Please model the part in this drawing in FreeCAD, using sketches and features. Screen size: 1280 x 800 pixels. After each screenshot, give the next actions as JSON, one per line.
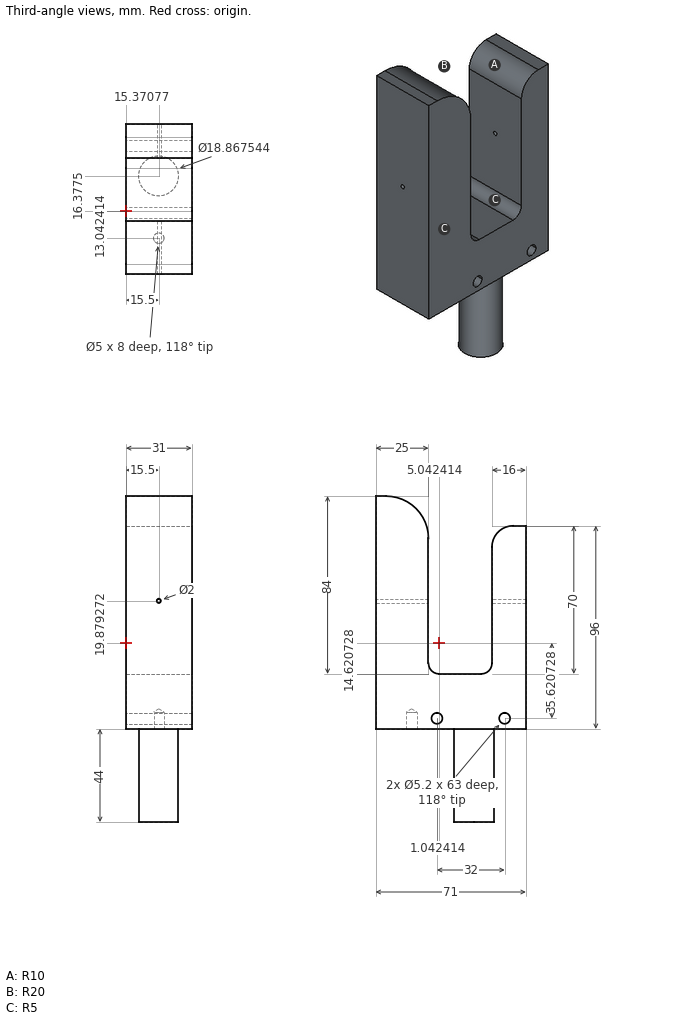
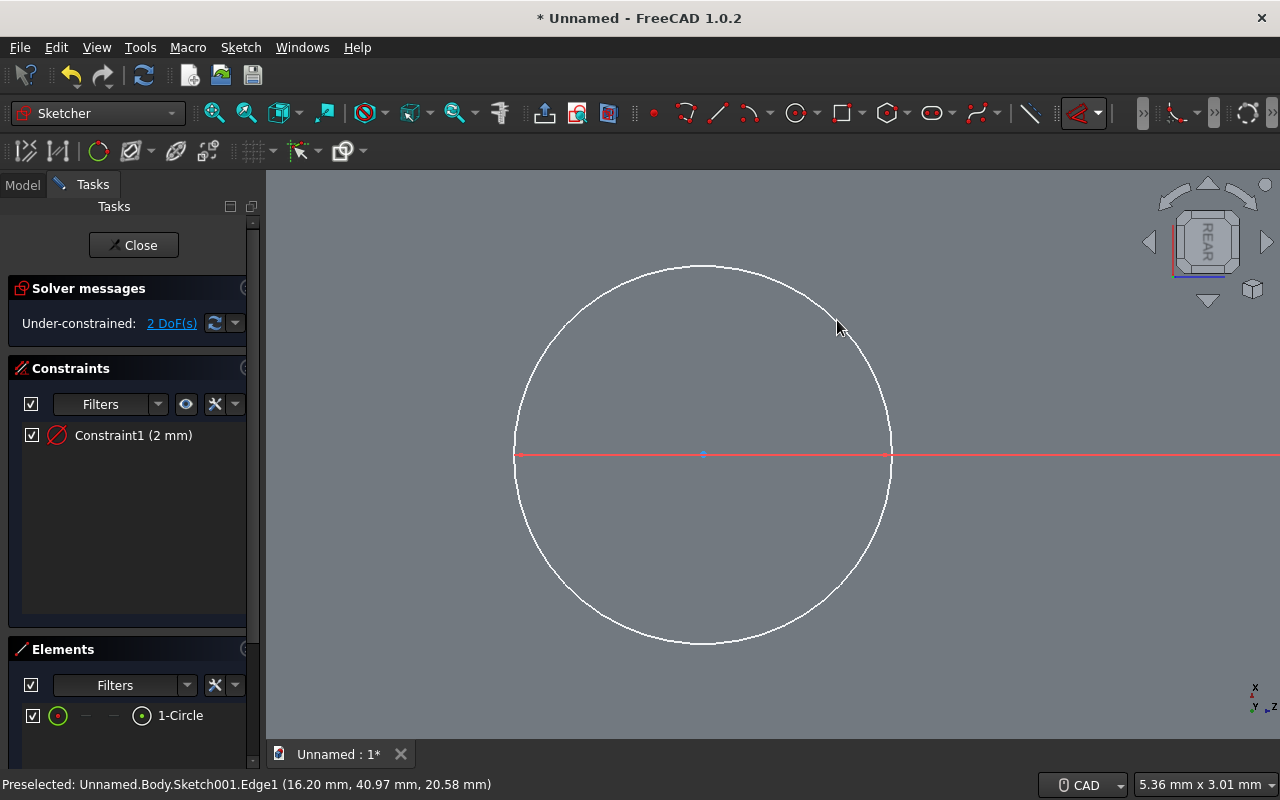
{"action": "left_click", "coordinate": [703, 455]}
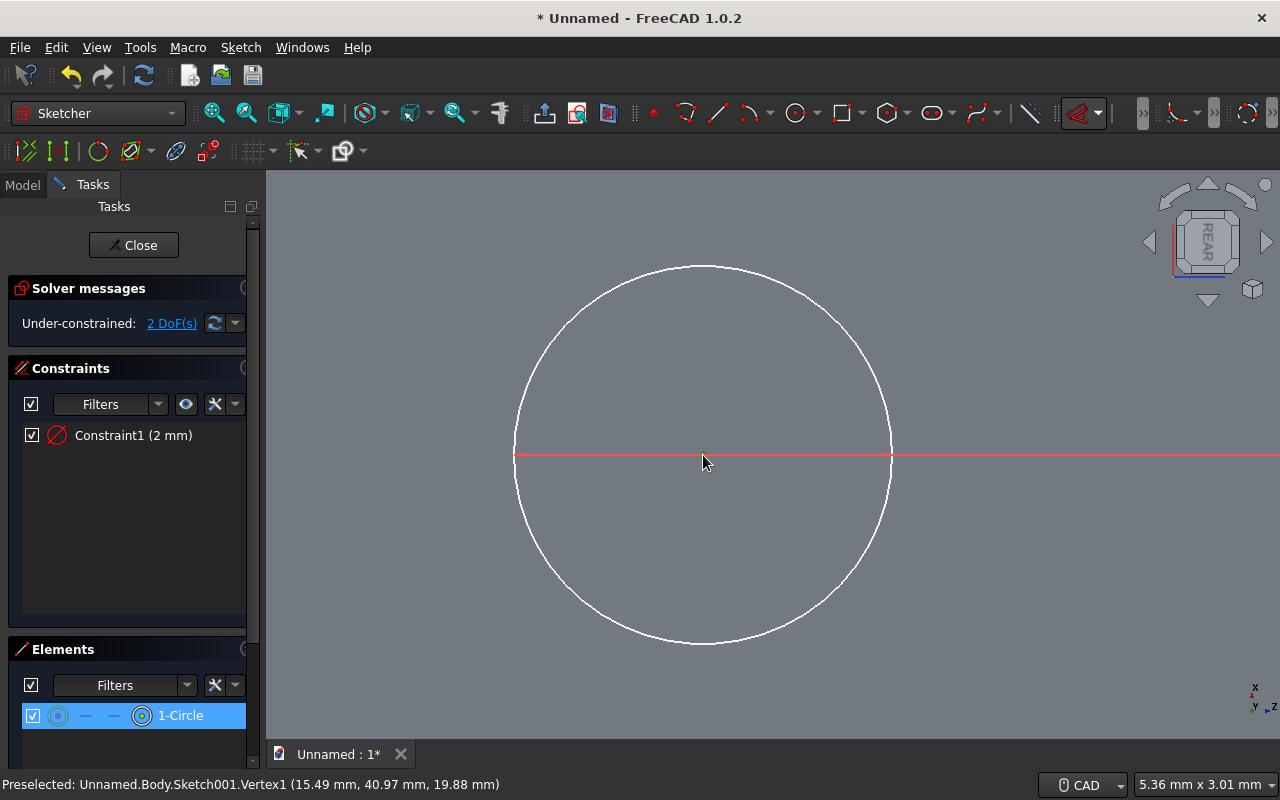
{"action": "left_click", "coordinate": [1100, 114]}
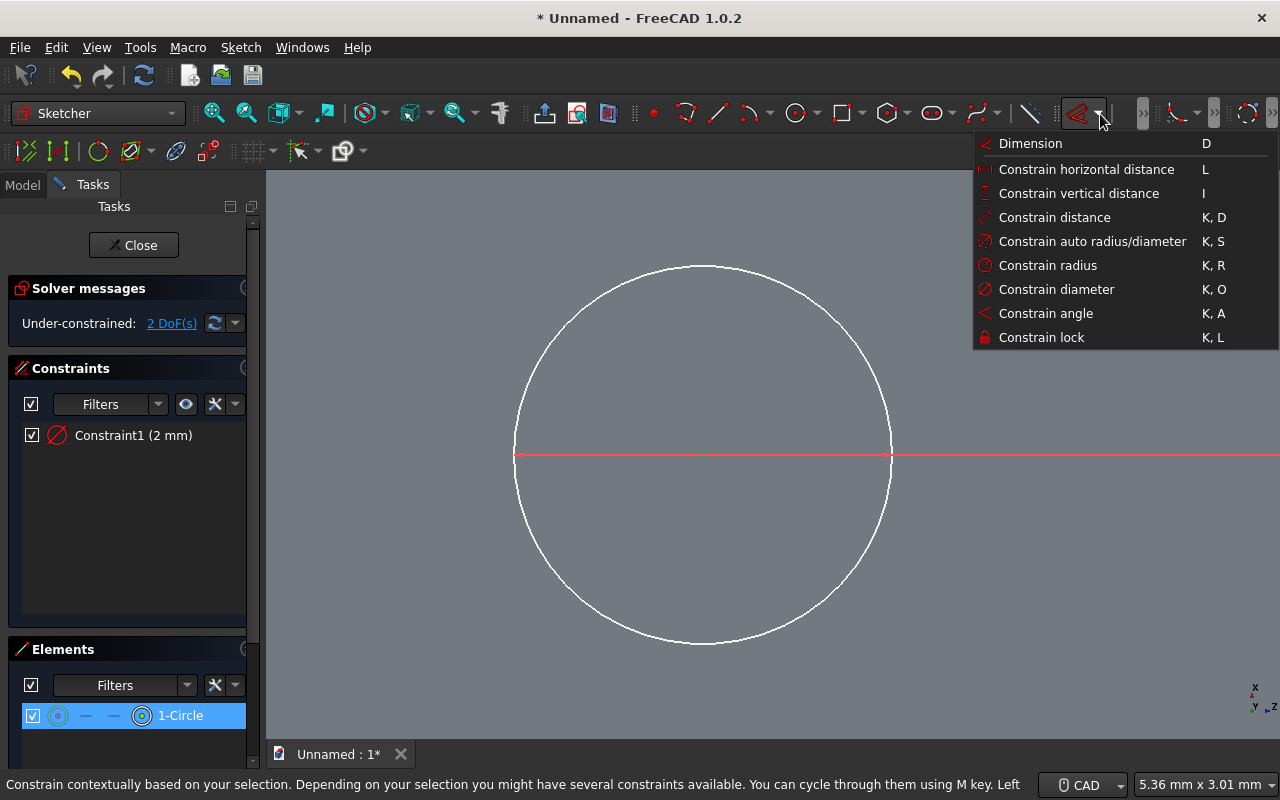
{"action": "left_click", "coordinate": [1126, 193]}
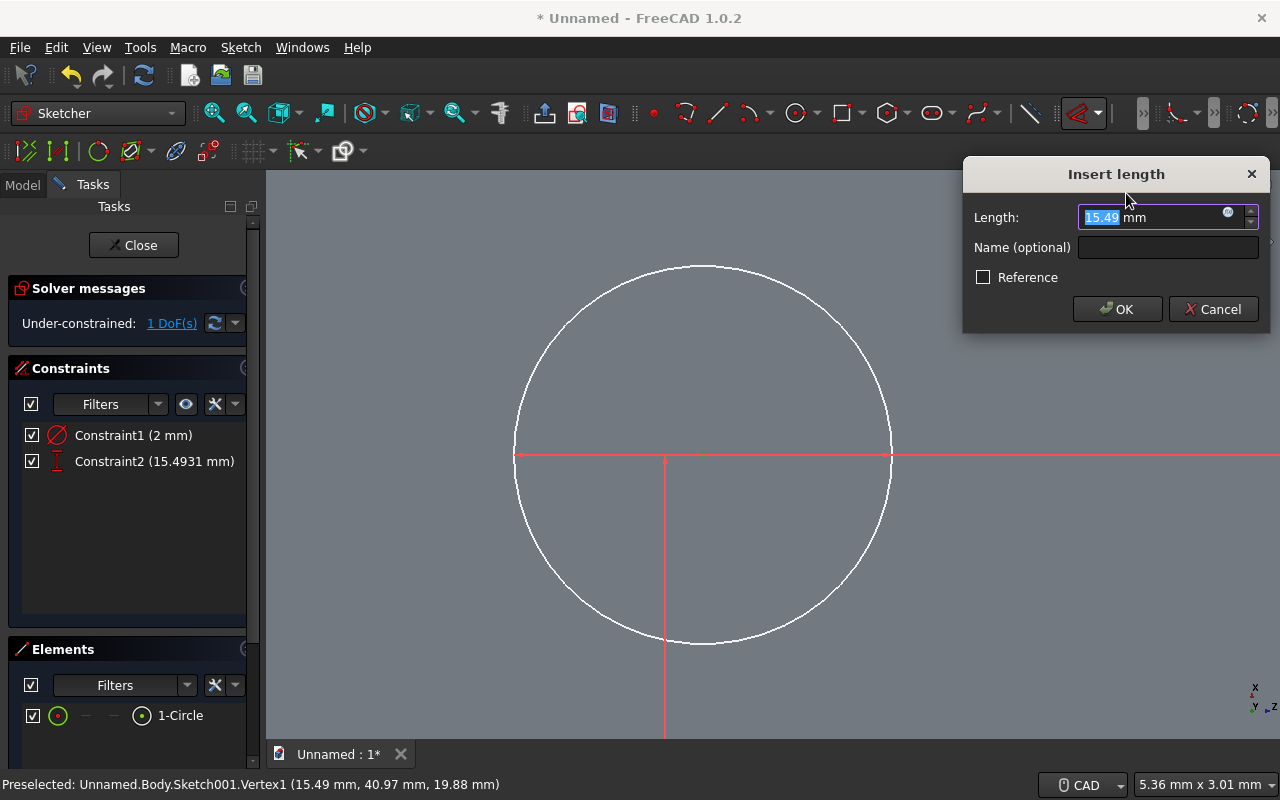
{"action": "type", "text": "15.5"}
{"action": "key", "text": "Return"}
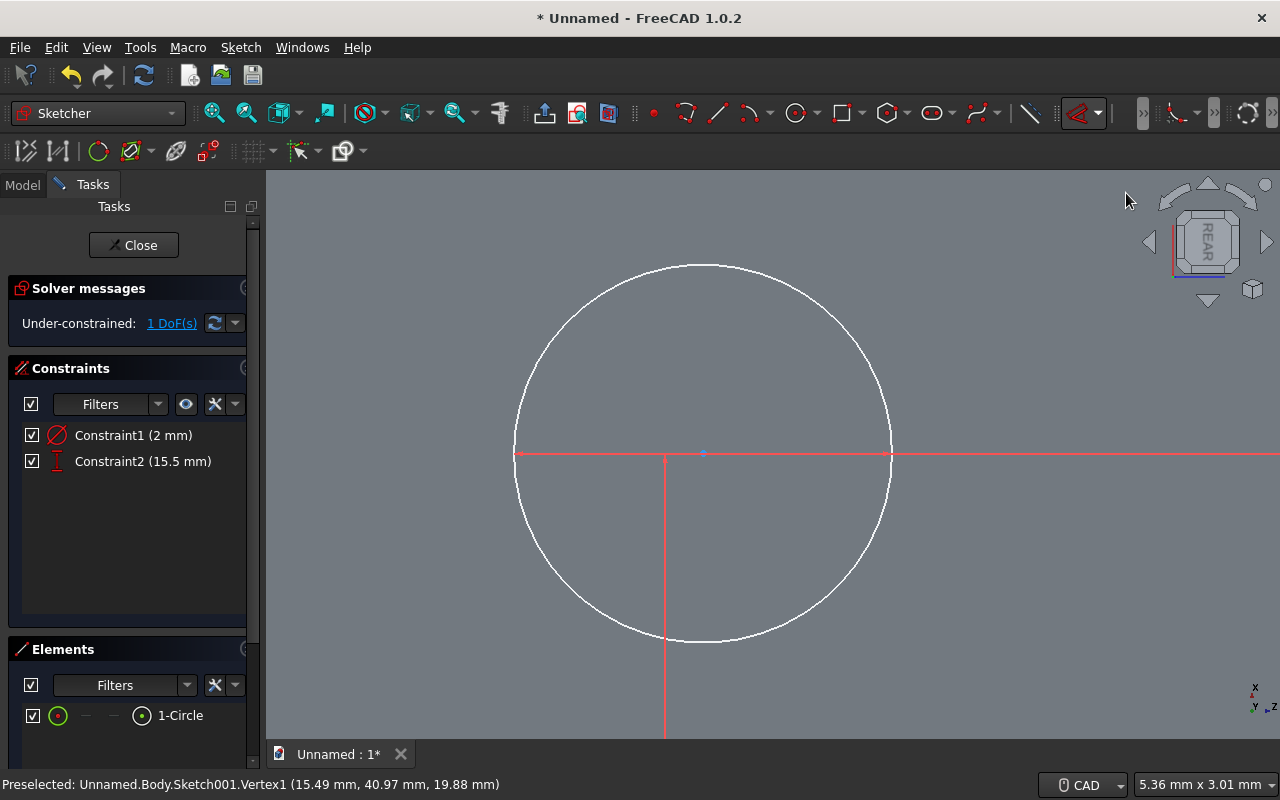
{"action": "left_click", "coordinate": [703, 454]}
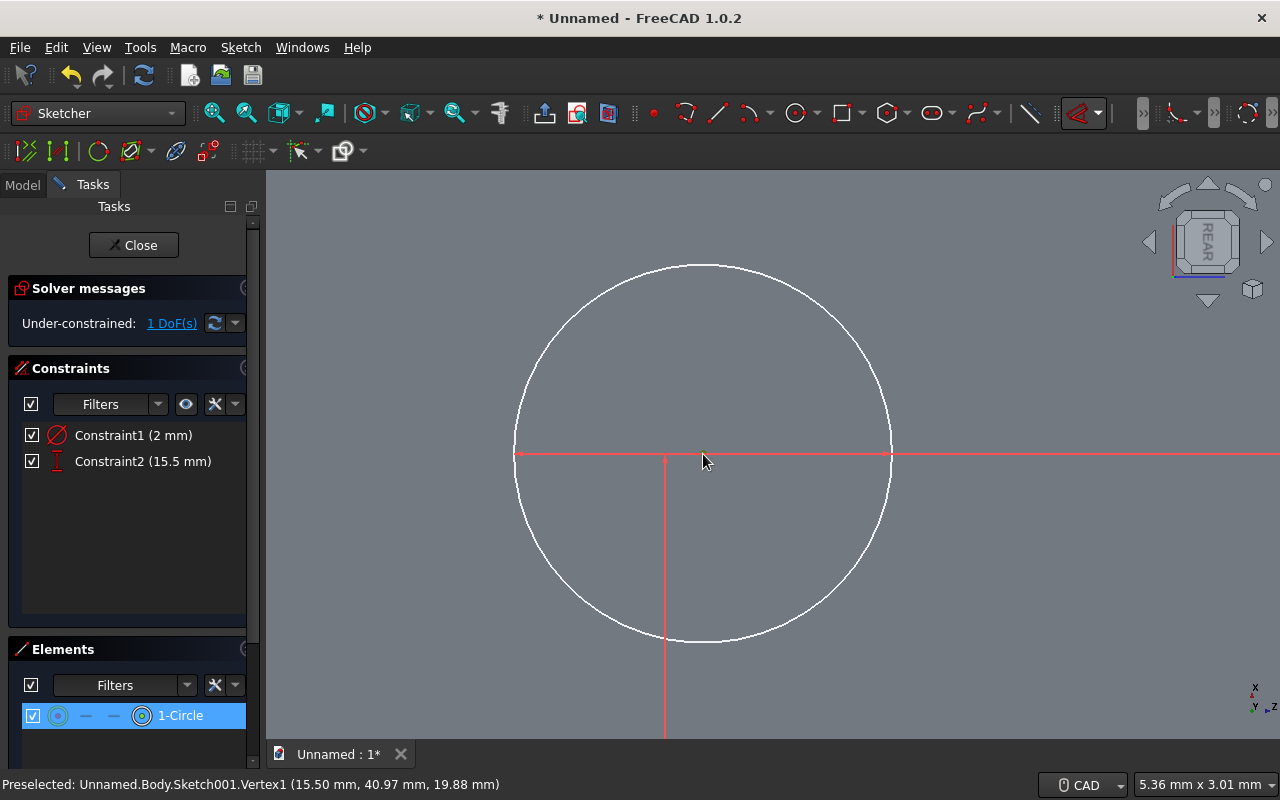
{"action": "key", "text": "l"}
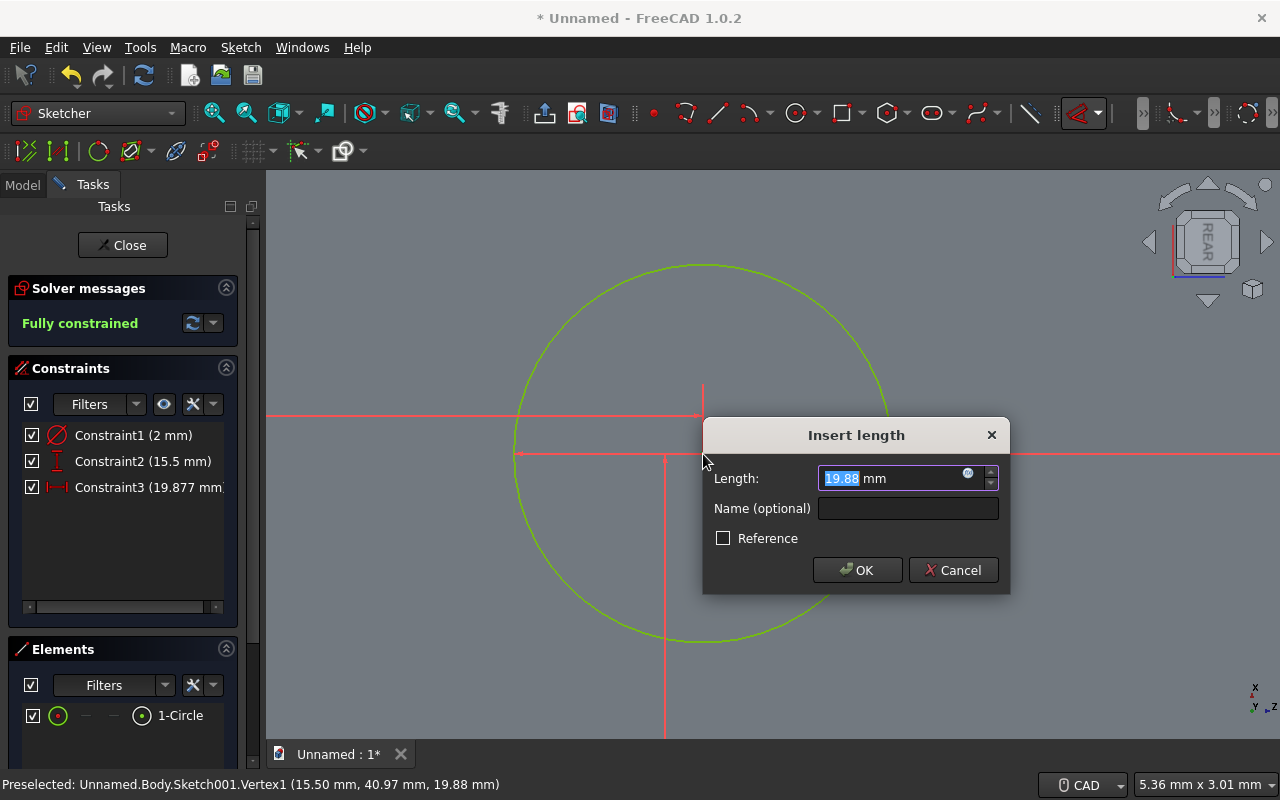
{"action": "type", "text": "19.879272"}
{"action": "key", "text": "Return"}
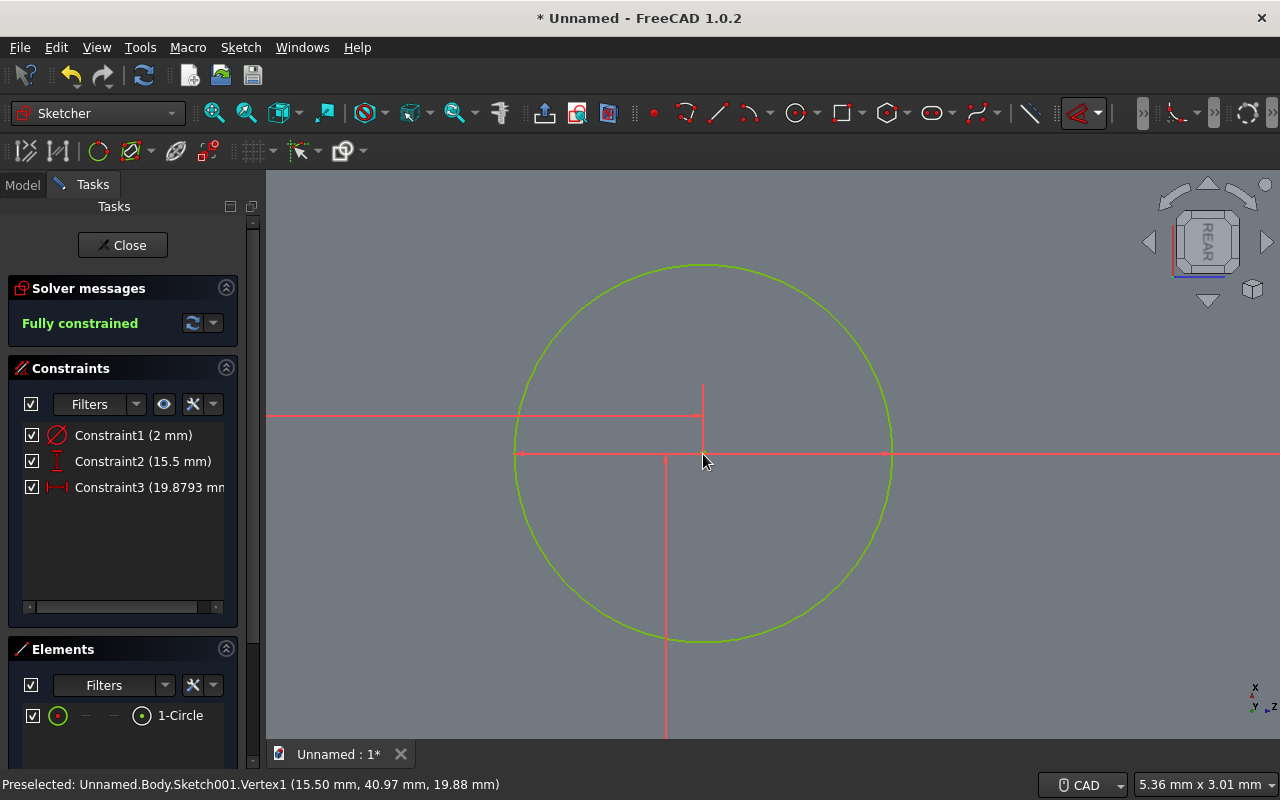
{"action": "left_click", "coordinate": [123, 245]}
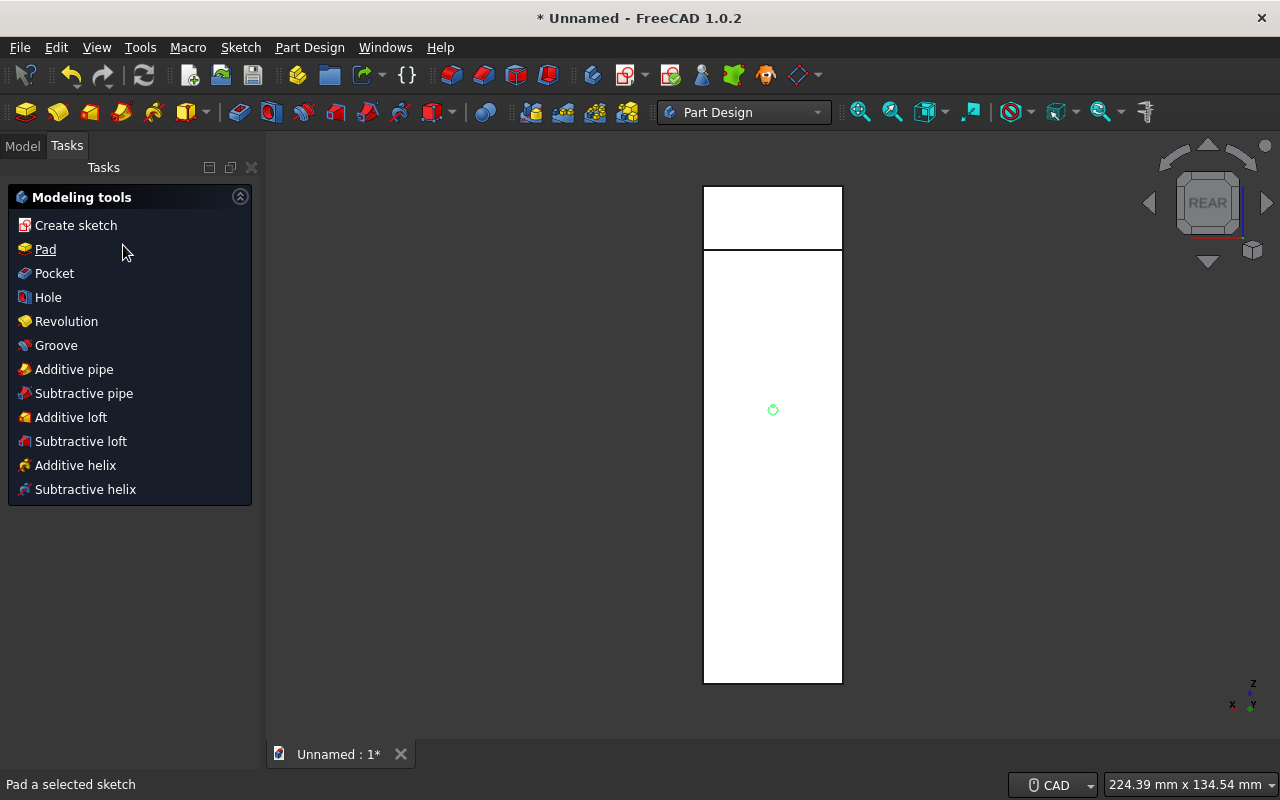
{"action": "left_click", "coordinate": [240, 112]}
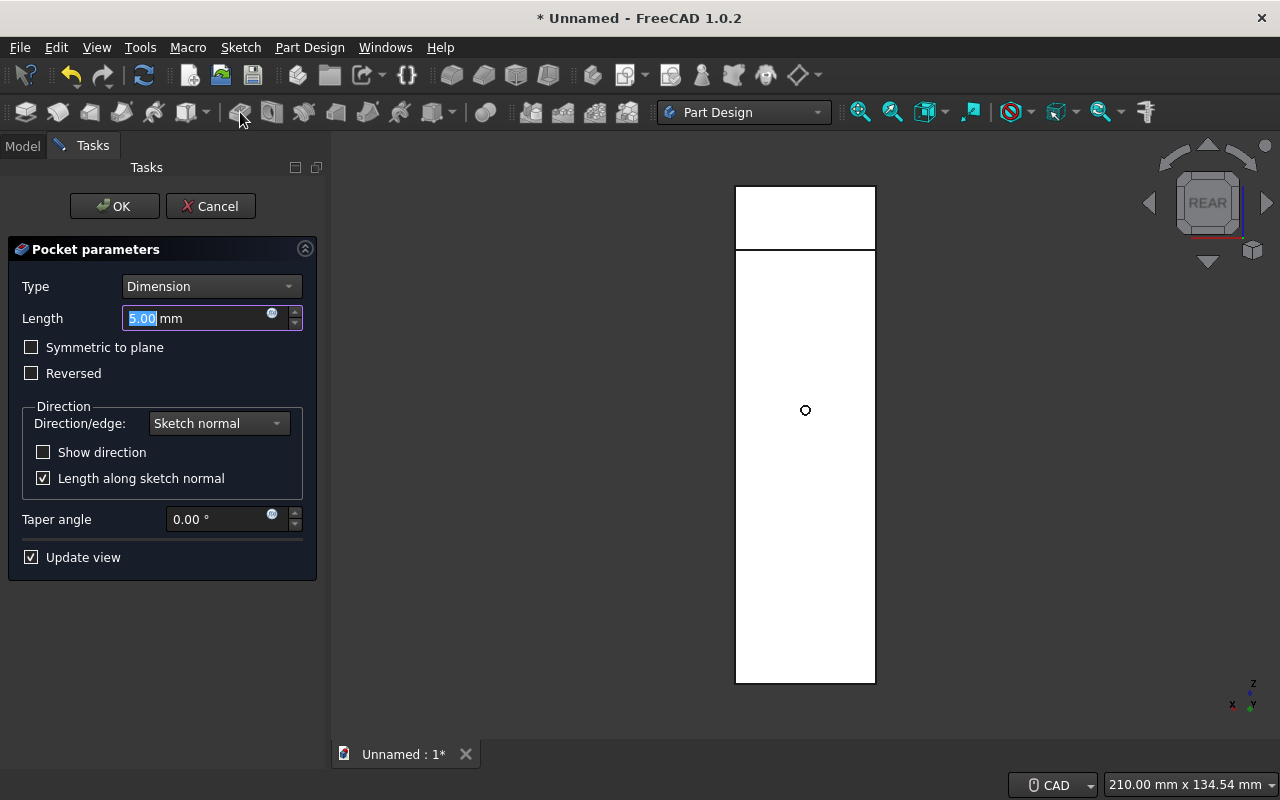
{"action": "left_click", "coordinate": [212, 286]}